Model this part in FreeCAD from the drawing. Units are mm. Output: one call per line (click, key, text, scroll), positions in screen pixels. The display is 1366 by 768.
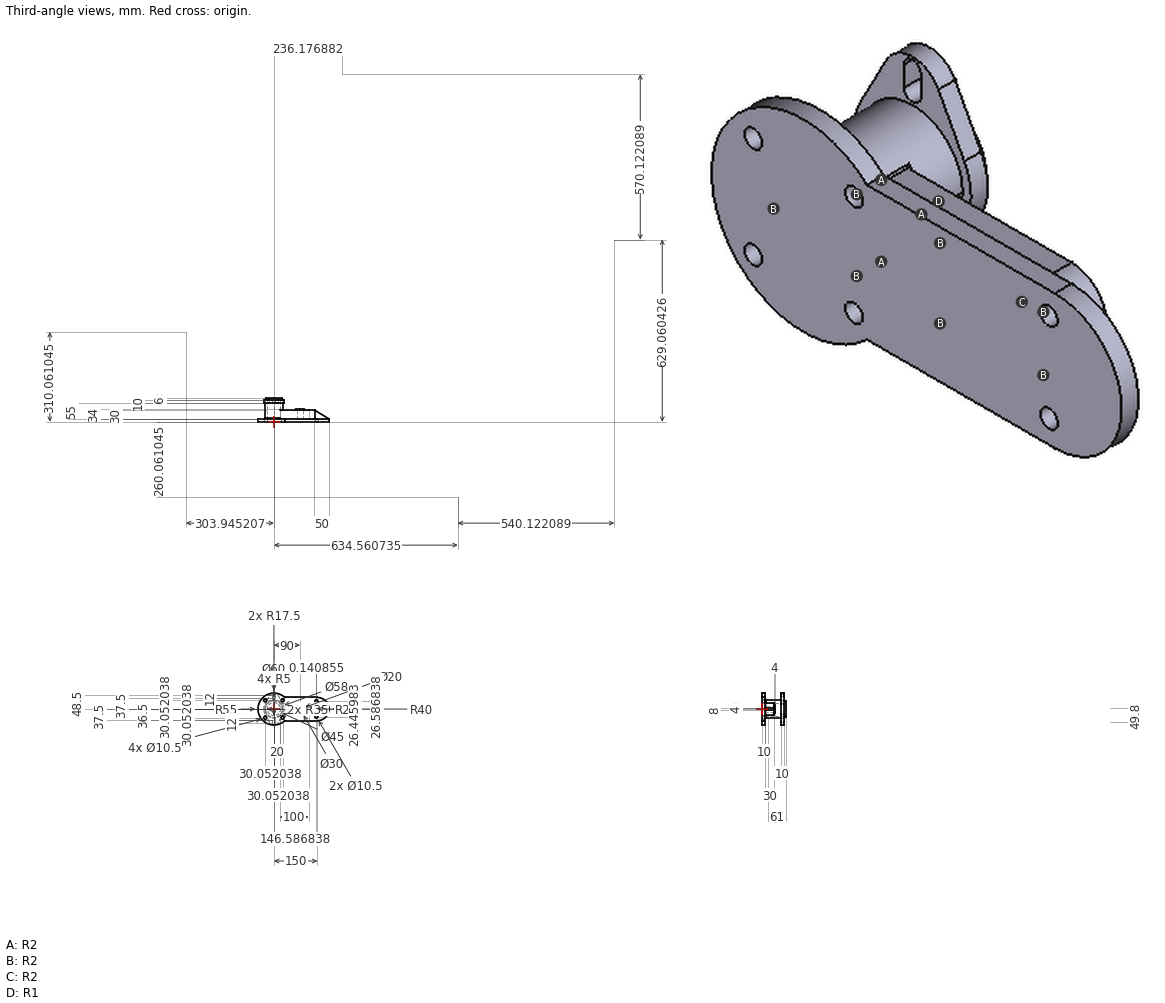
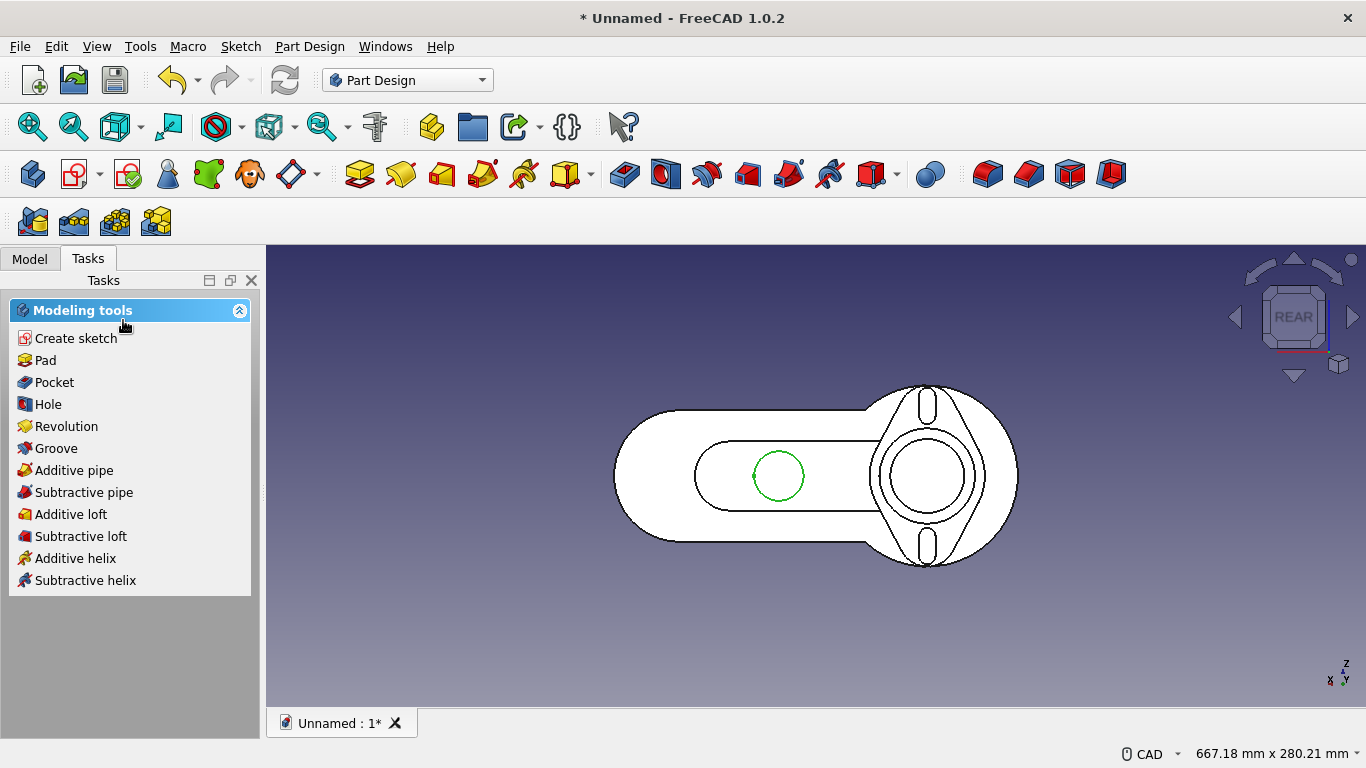
click(360, 174)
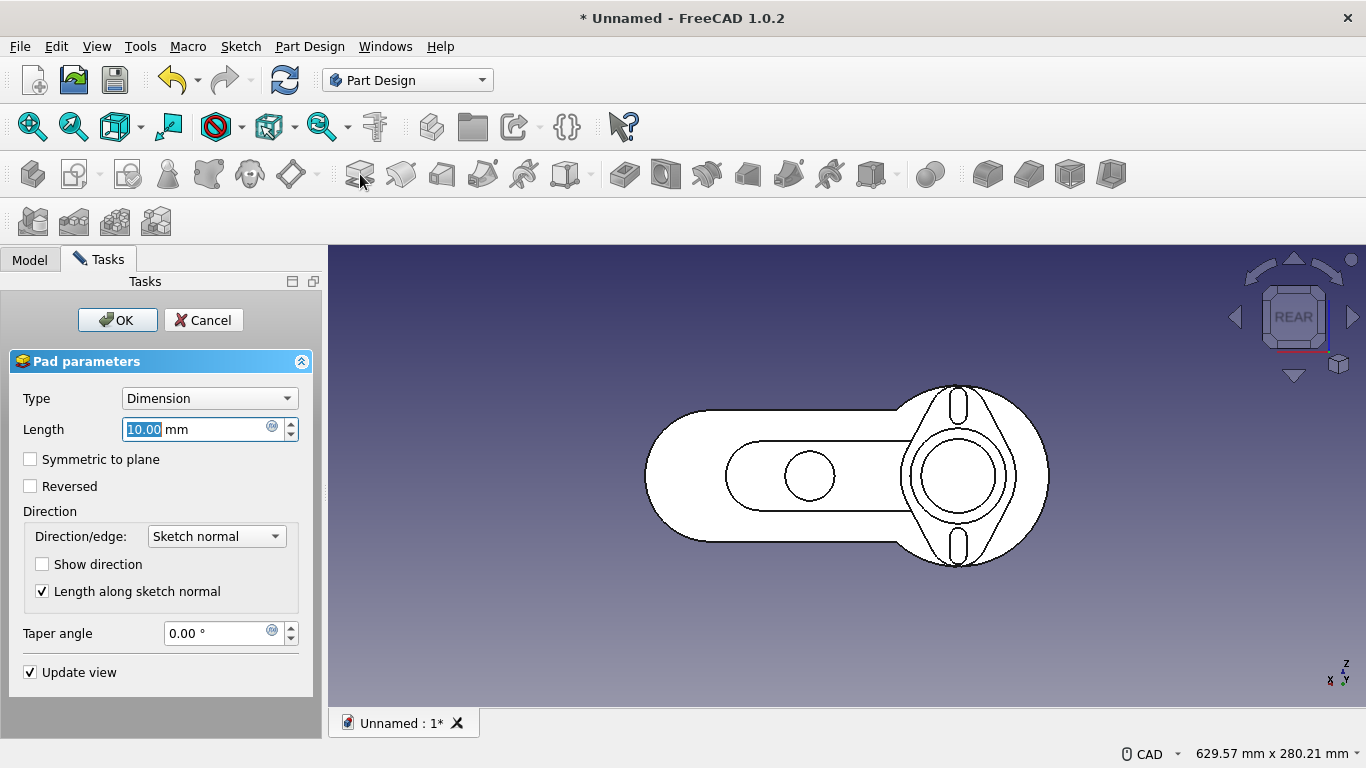
text(4)
key(Tab)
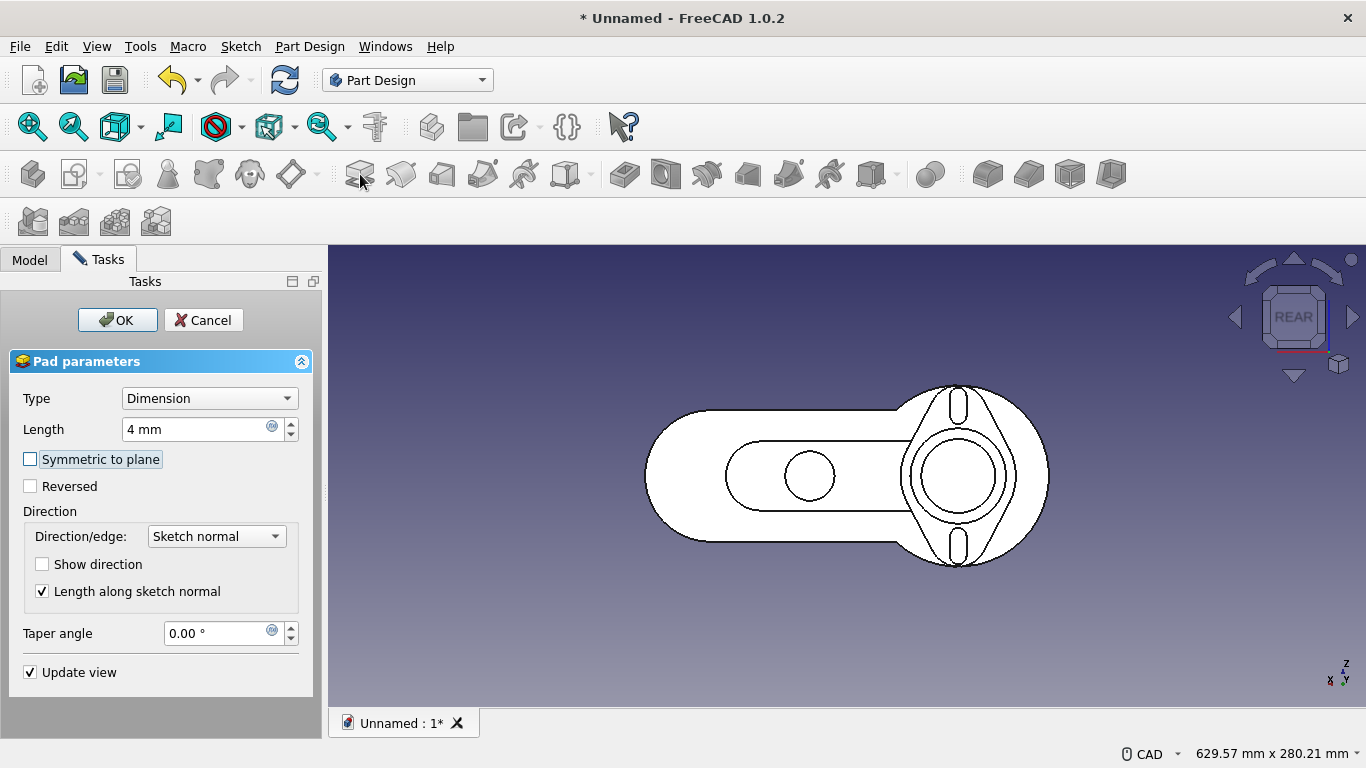
click(118, 320)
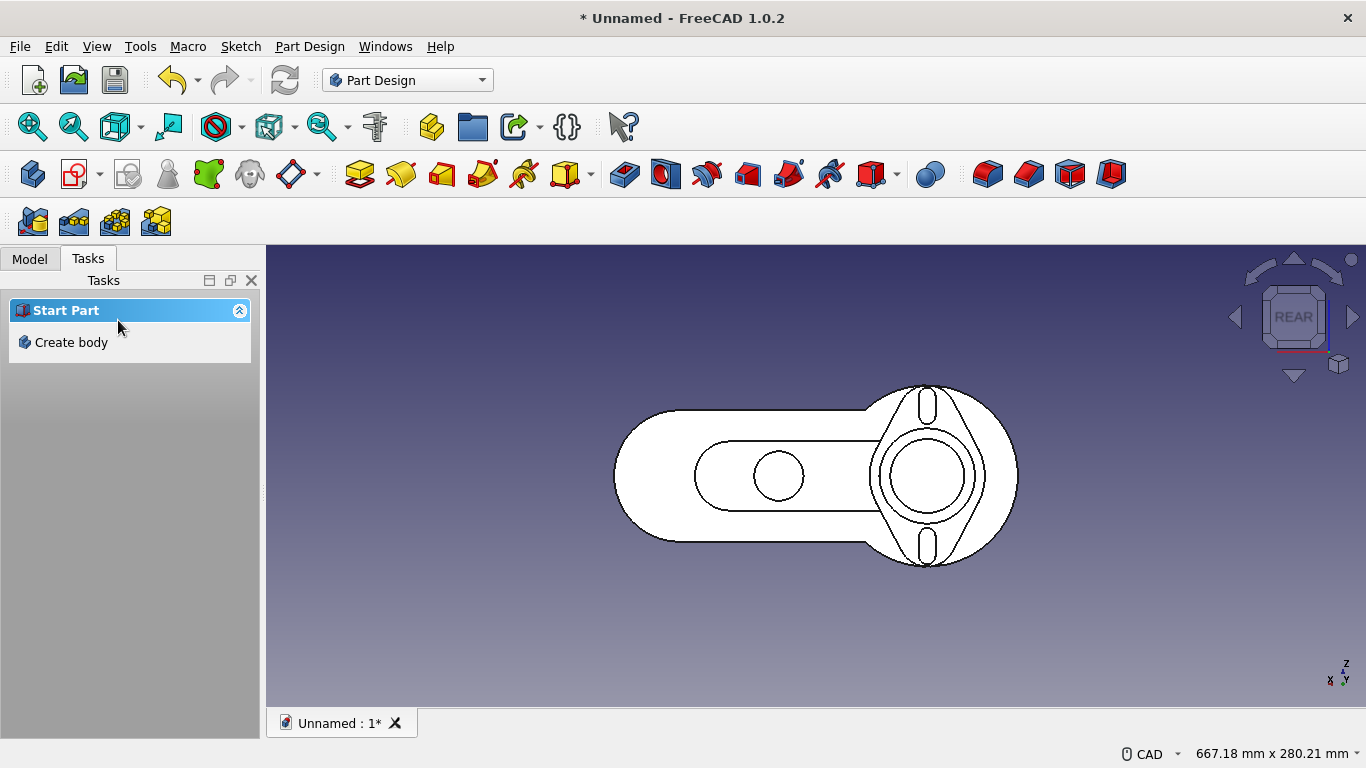
click(33, 128)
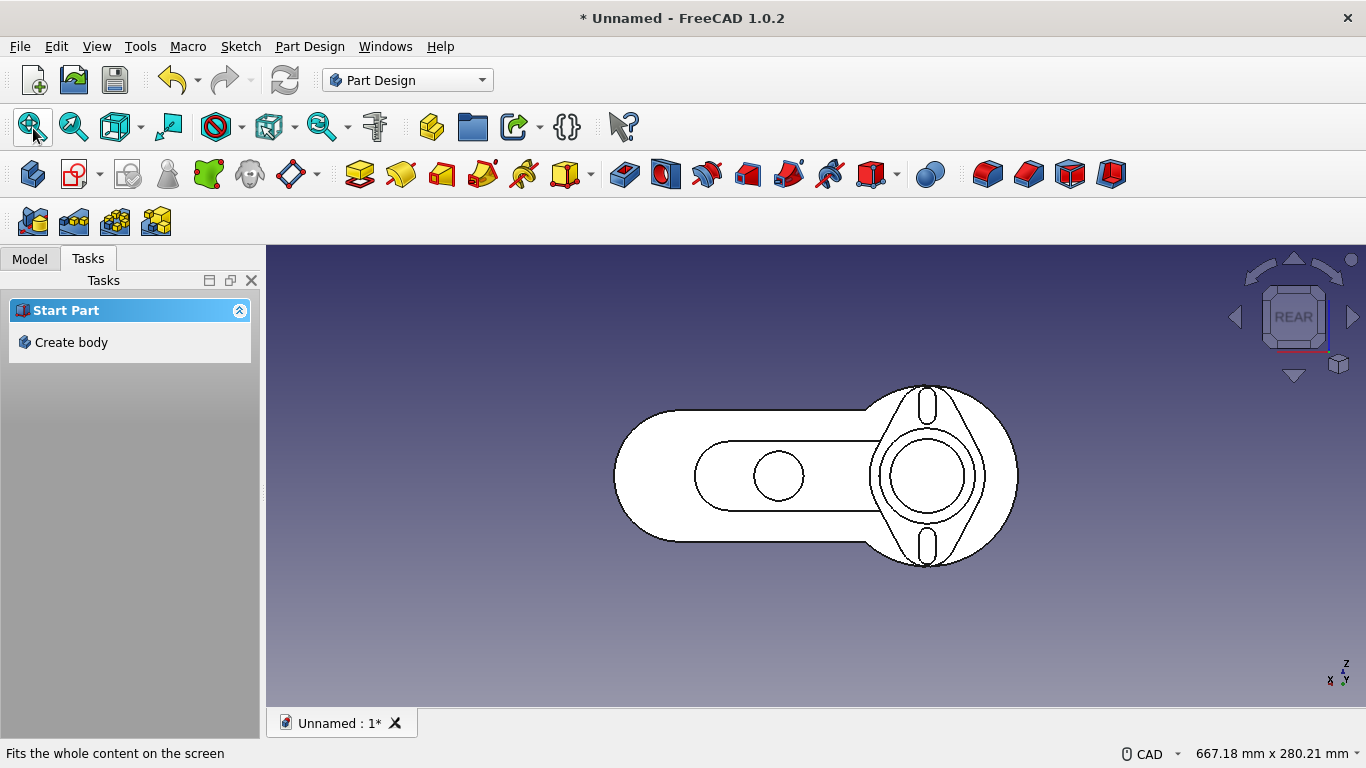
click(779, 475)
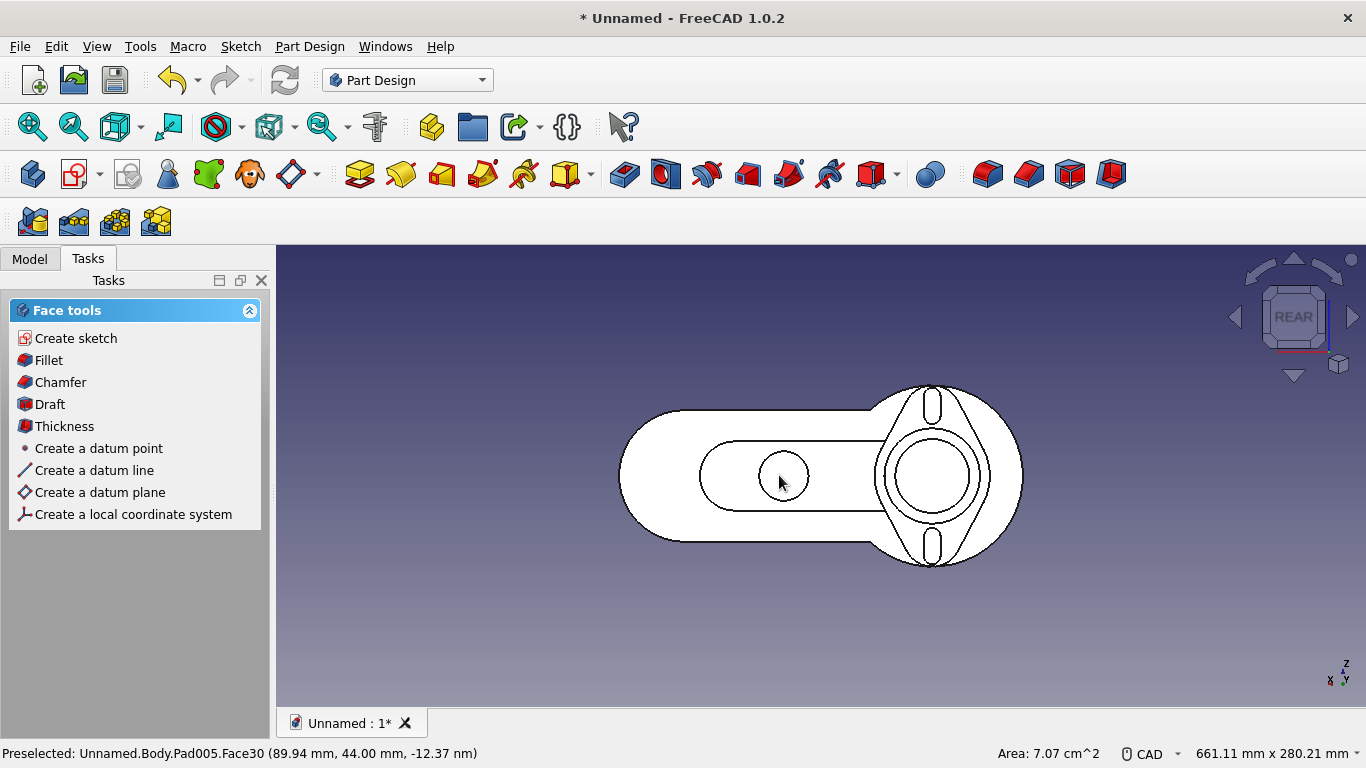
click(74, 174)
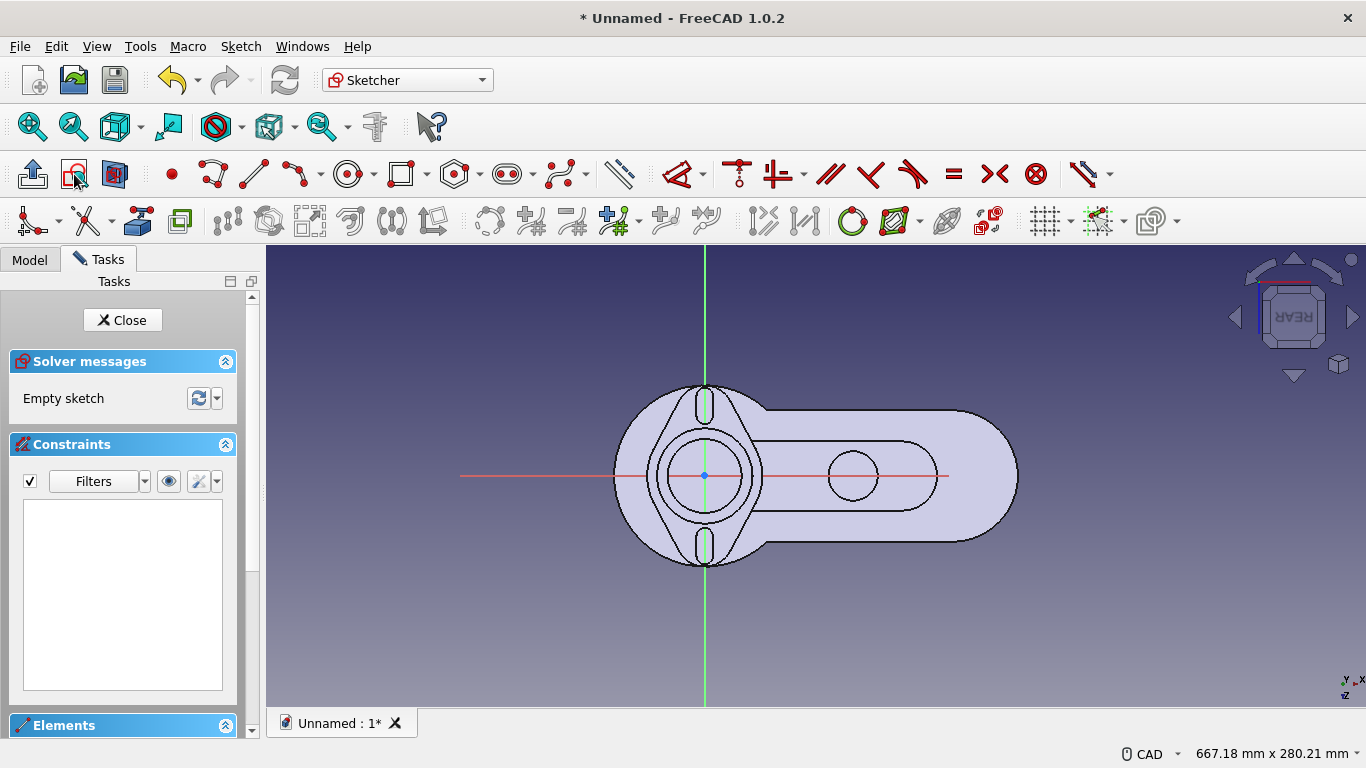
scroll(866, 476, up, 11)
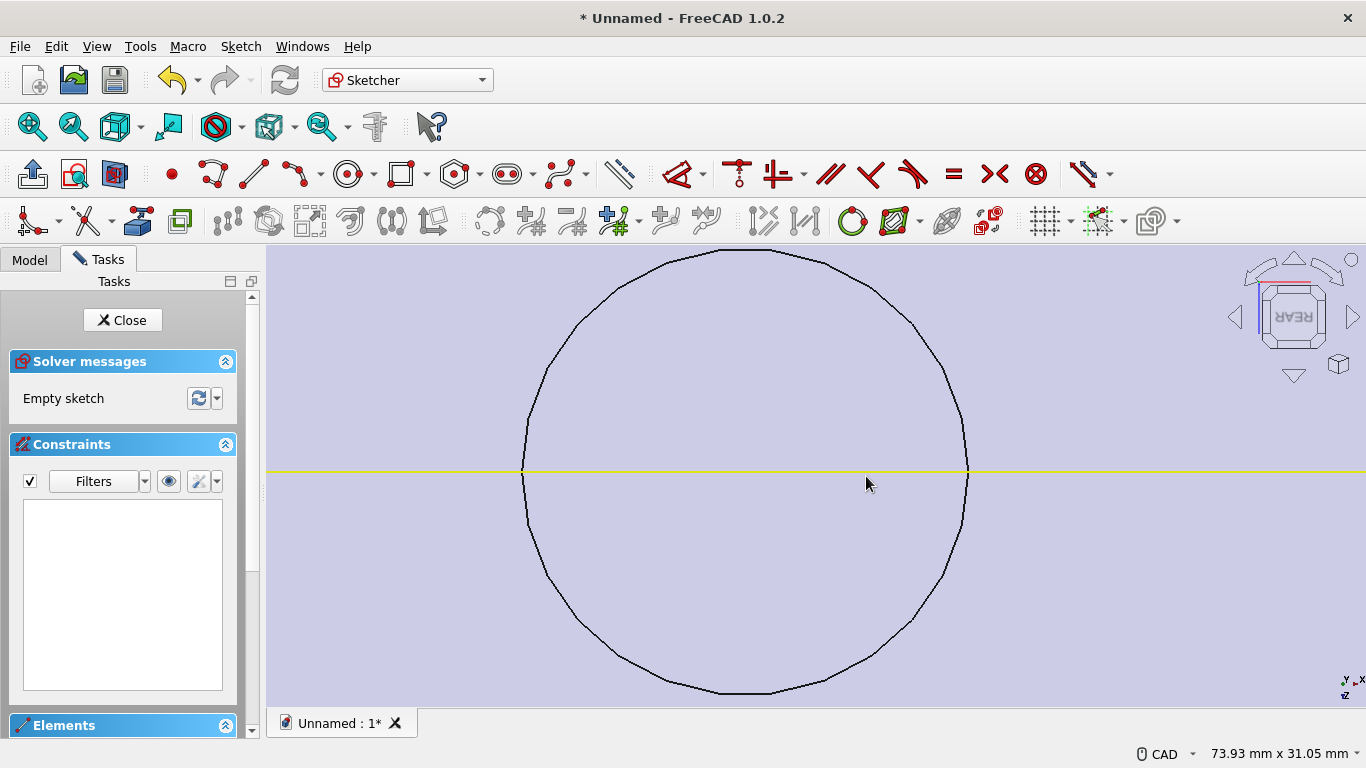
click(348, 174)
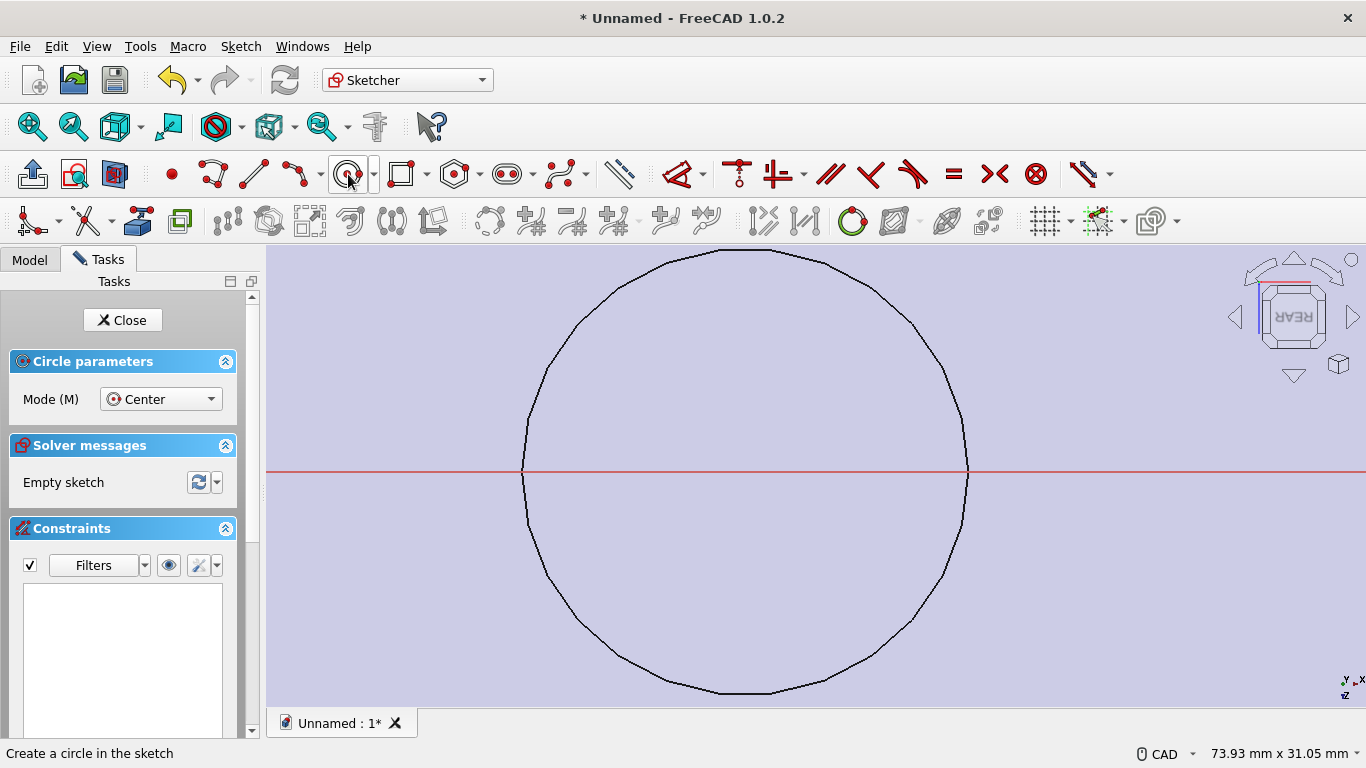
click(745, 472)
click(850, 367)
key(Escape)